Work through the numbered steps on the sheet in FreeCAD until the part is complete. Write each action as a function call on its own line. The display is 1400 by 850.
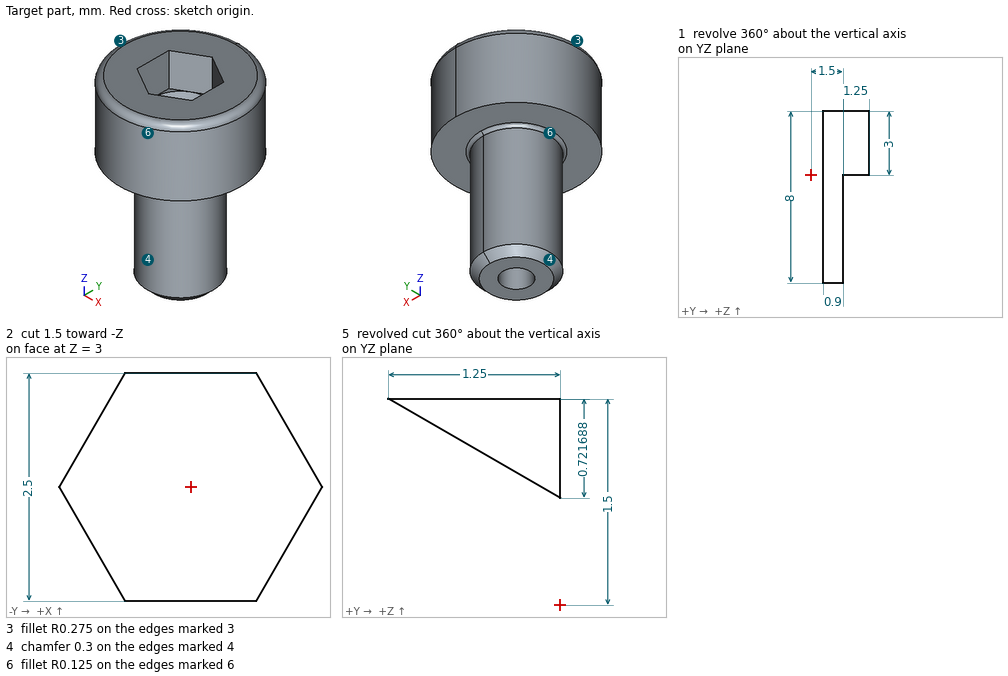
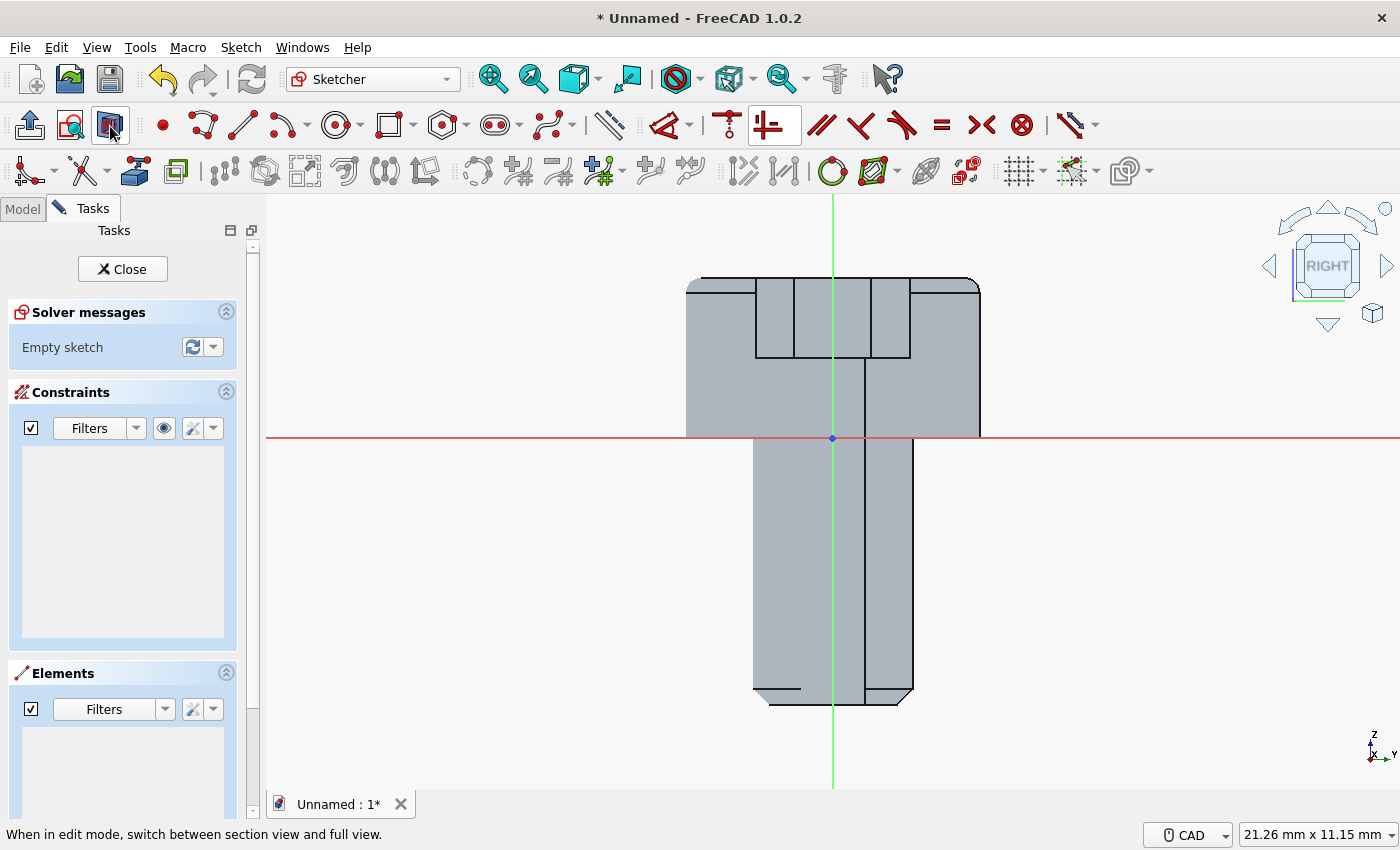
scroll(808, 375, up, 8)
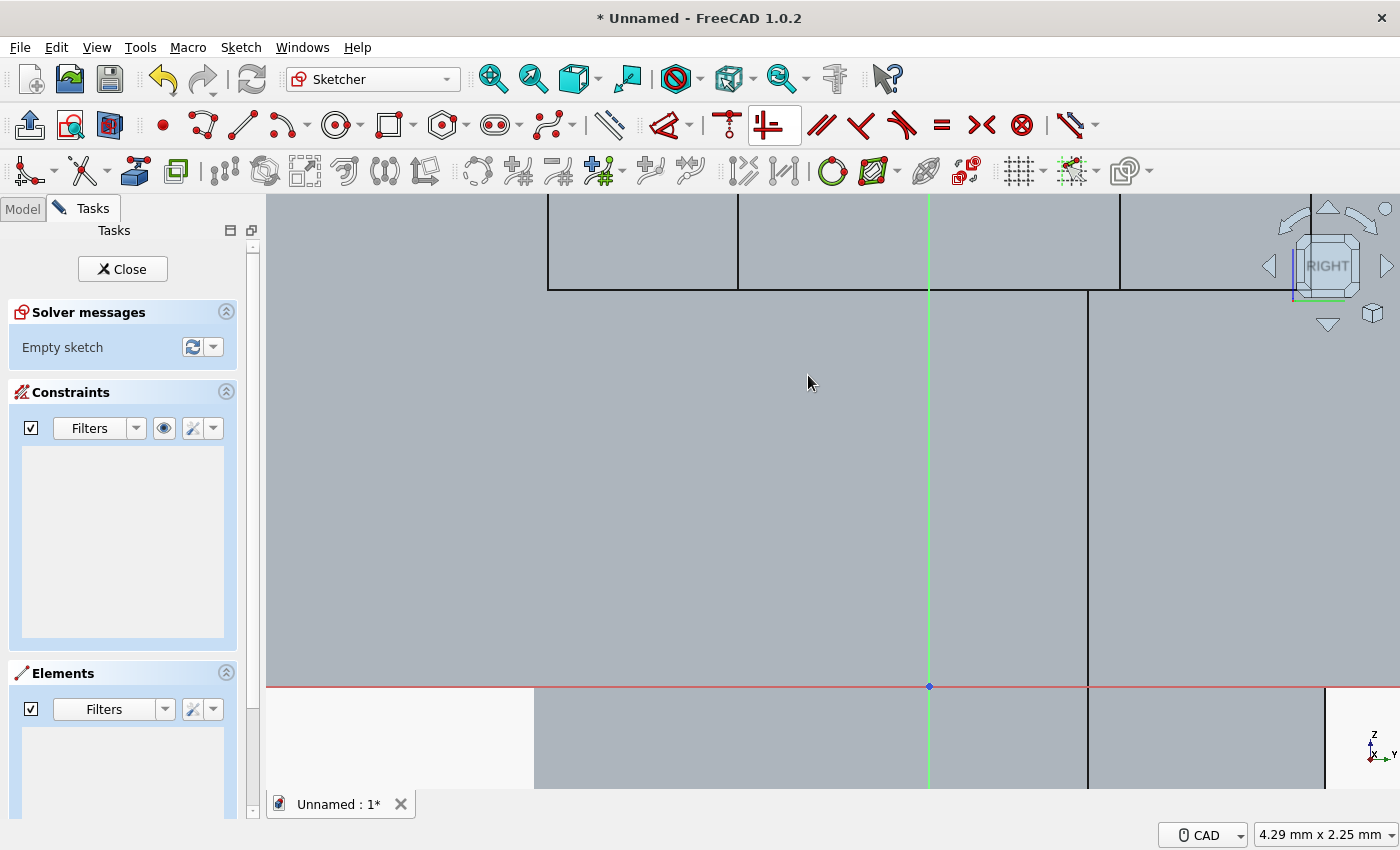
click(204, 126)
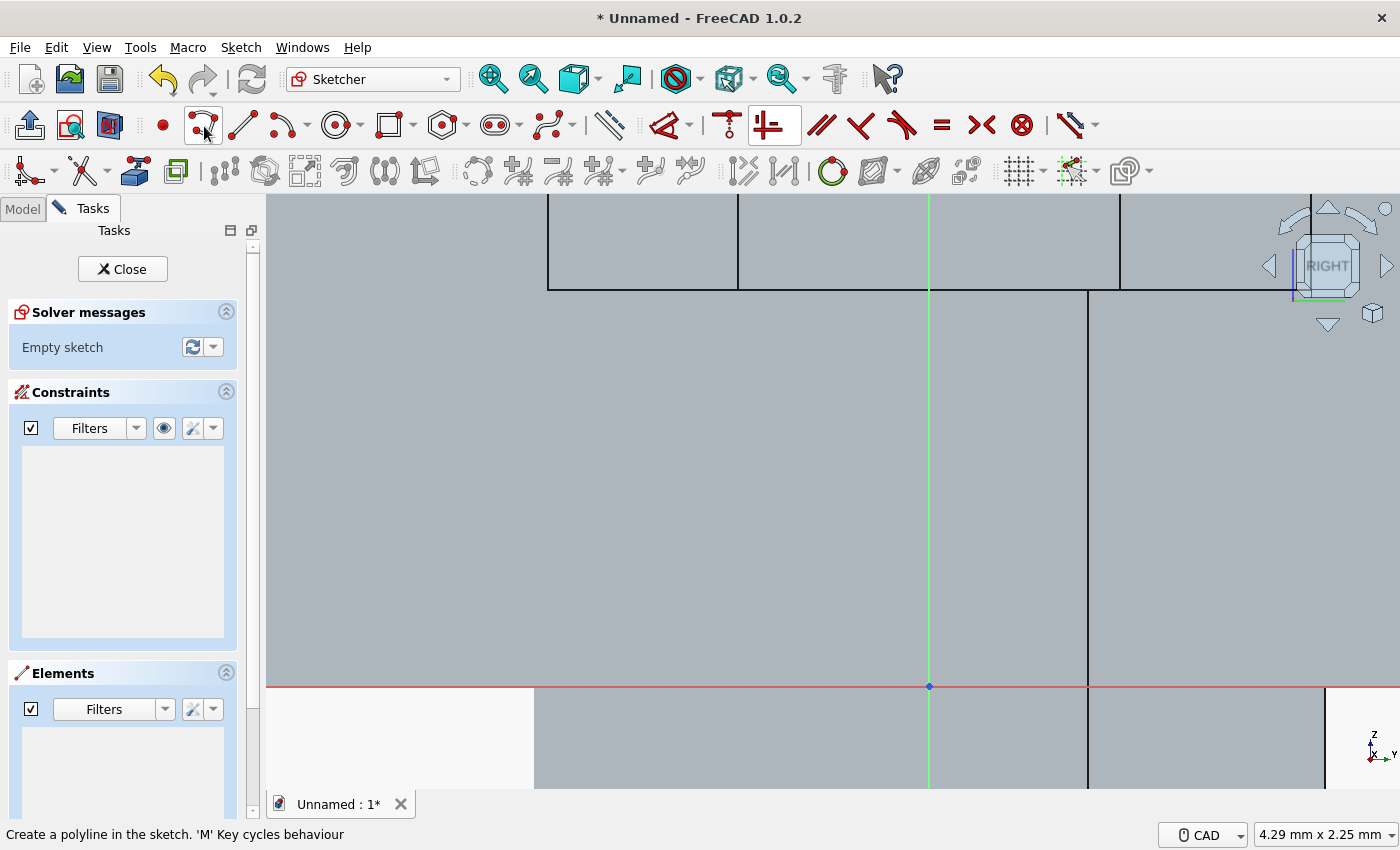
click(929, 481)
click(920, 290)
click(599, 290)
click(929, 482)
key(Escape)
key(Escape)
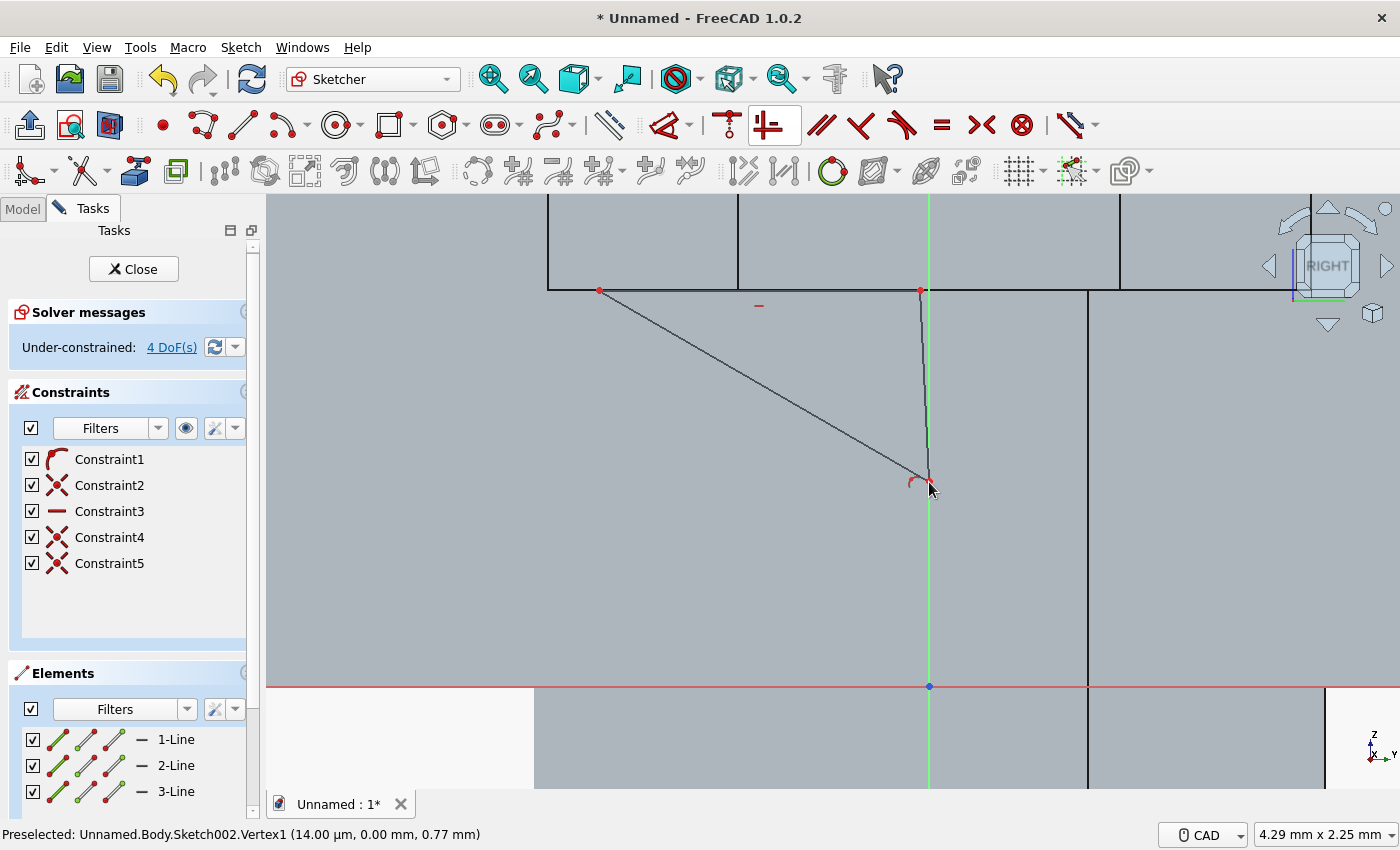
click(926, 425)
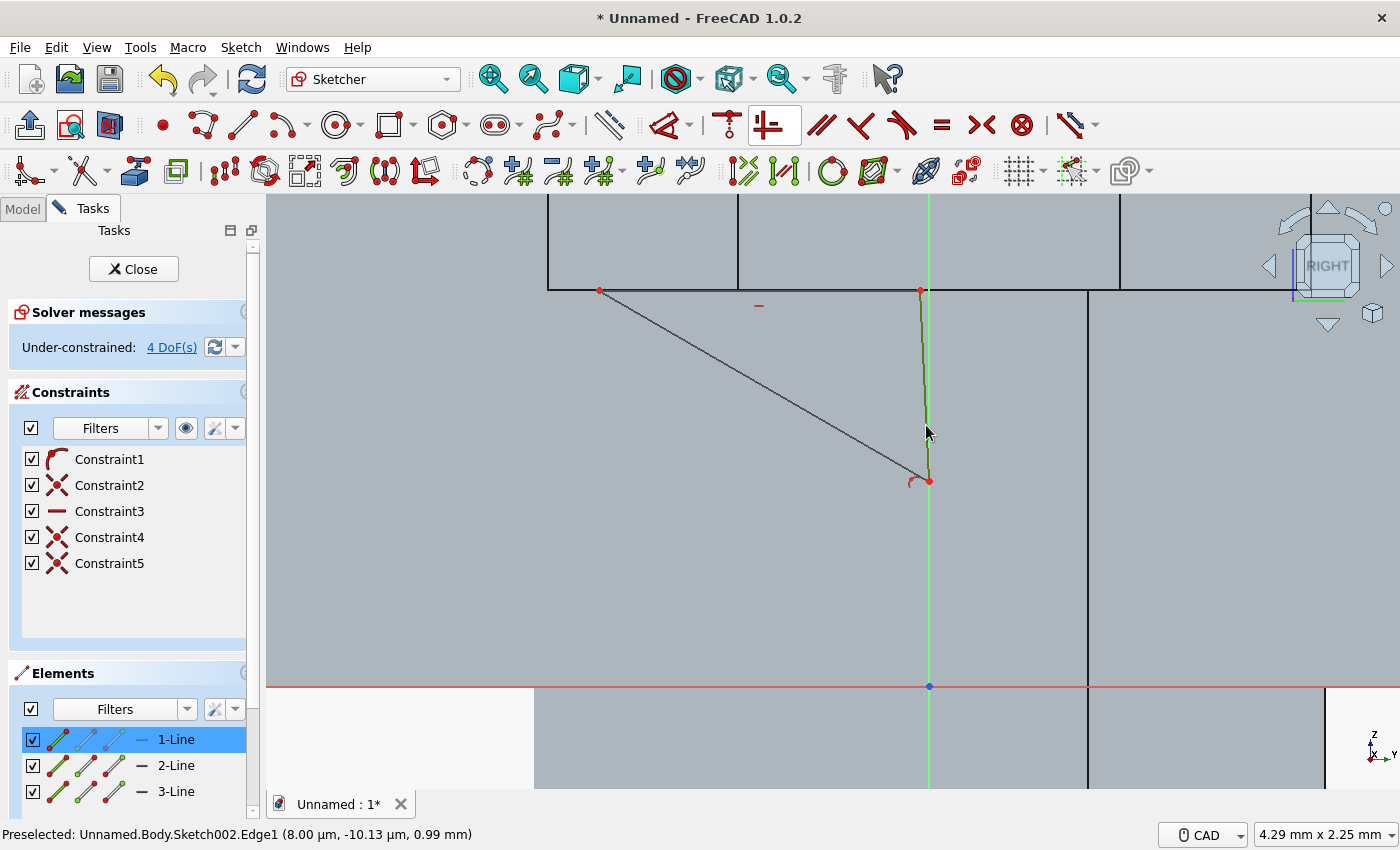
click(796, 126)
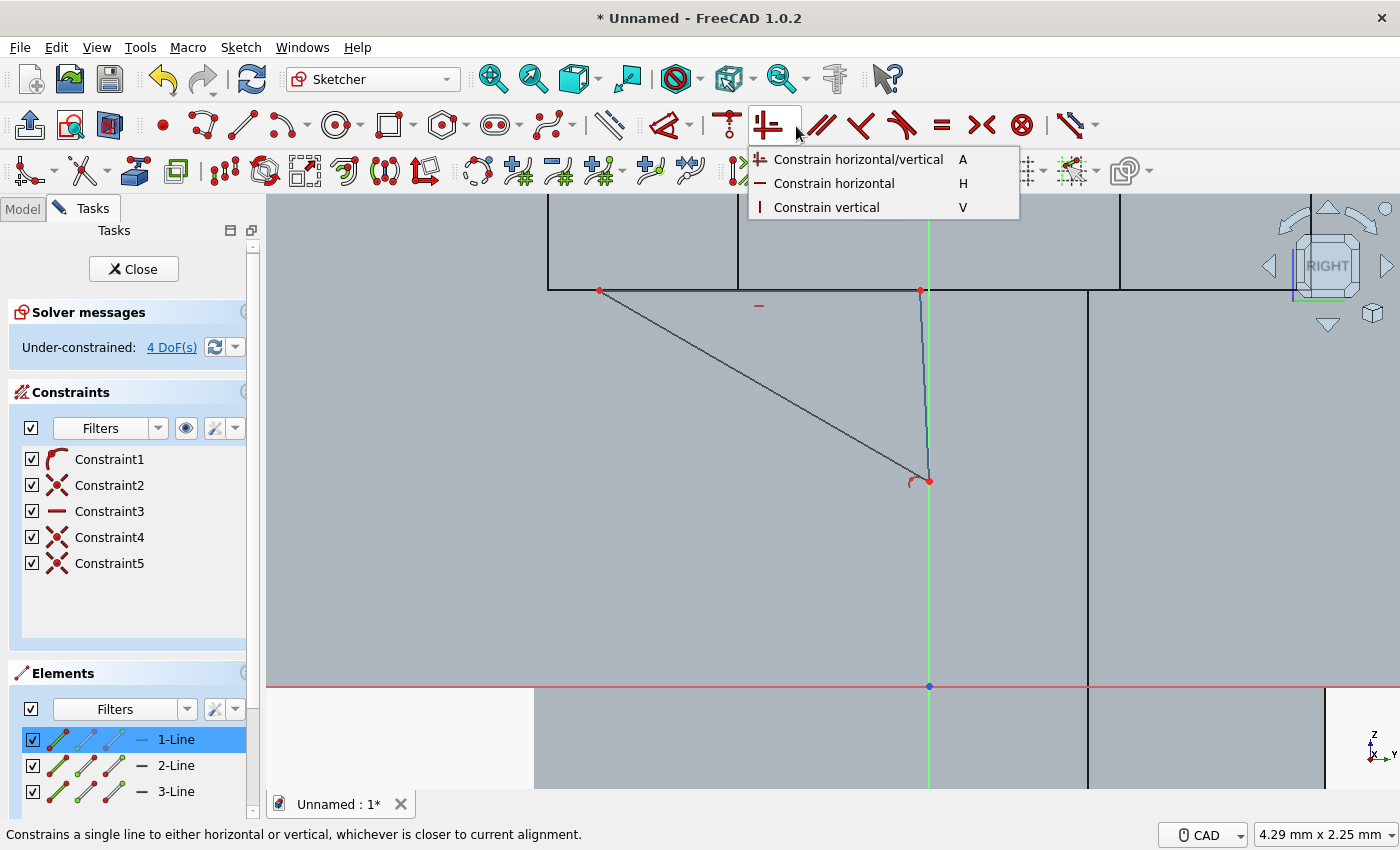
click(884, 207)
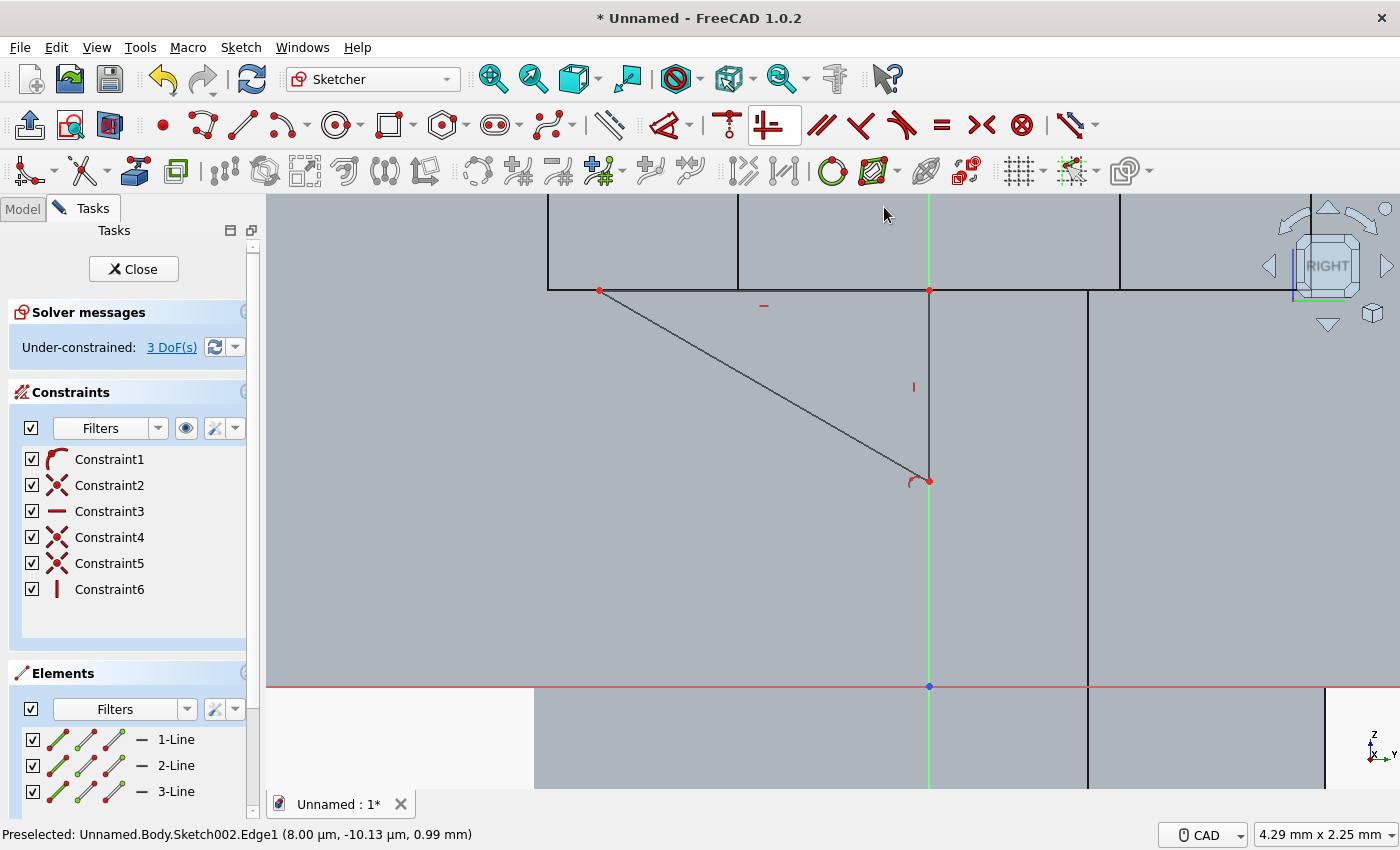
click(664, 126)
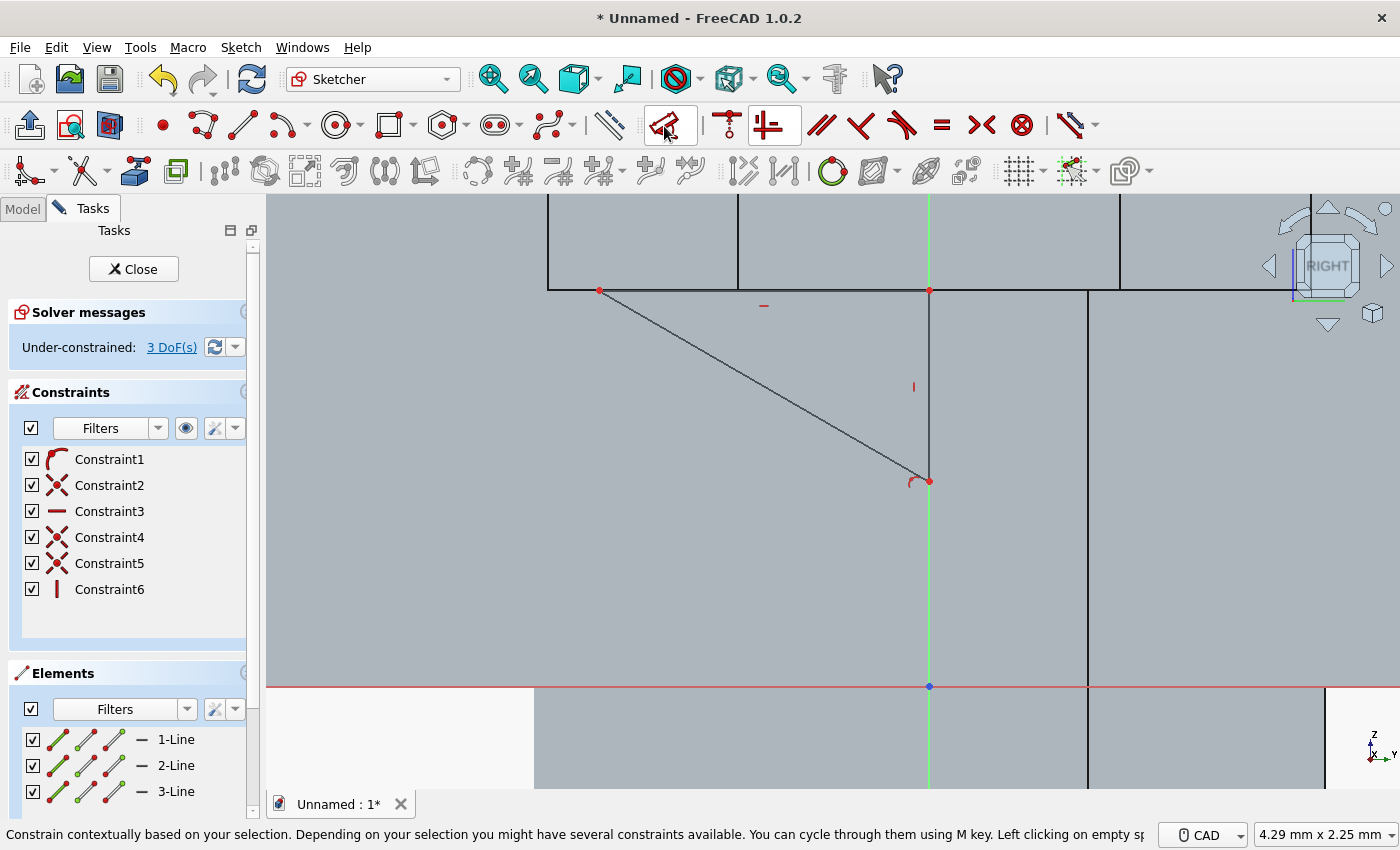
click(830, 291)
click(764, 257)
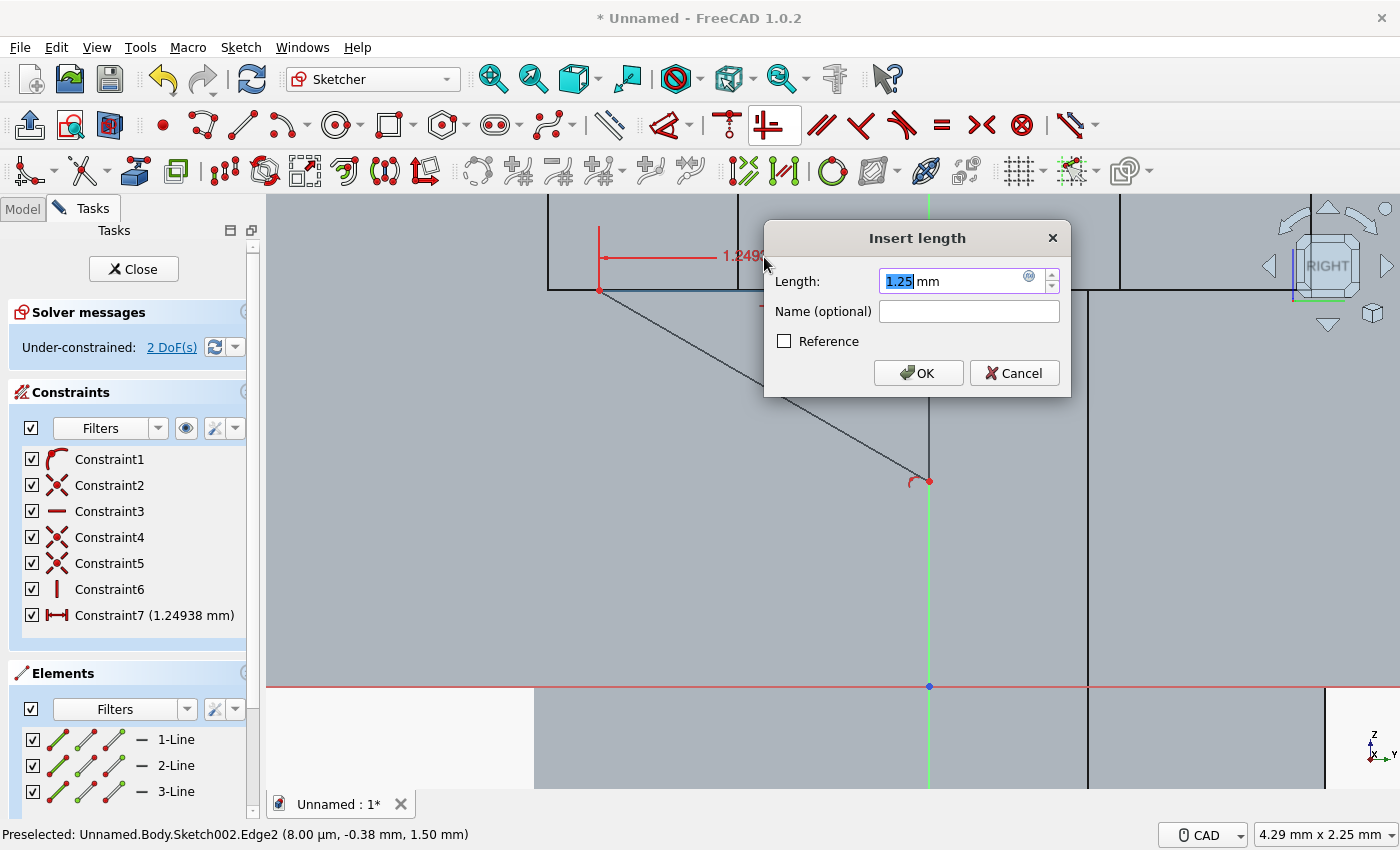
text(1.25)
key(Return)